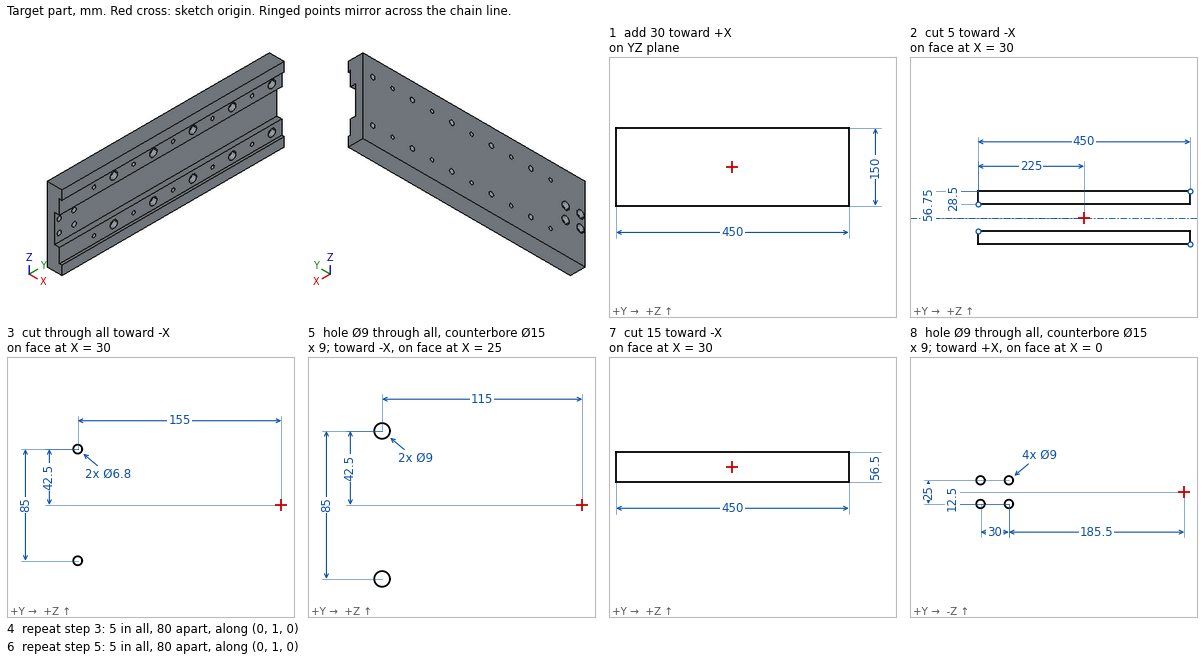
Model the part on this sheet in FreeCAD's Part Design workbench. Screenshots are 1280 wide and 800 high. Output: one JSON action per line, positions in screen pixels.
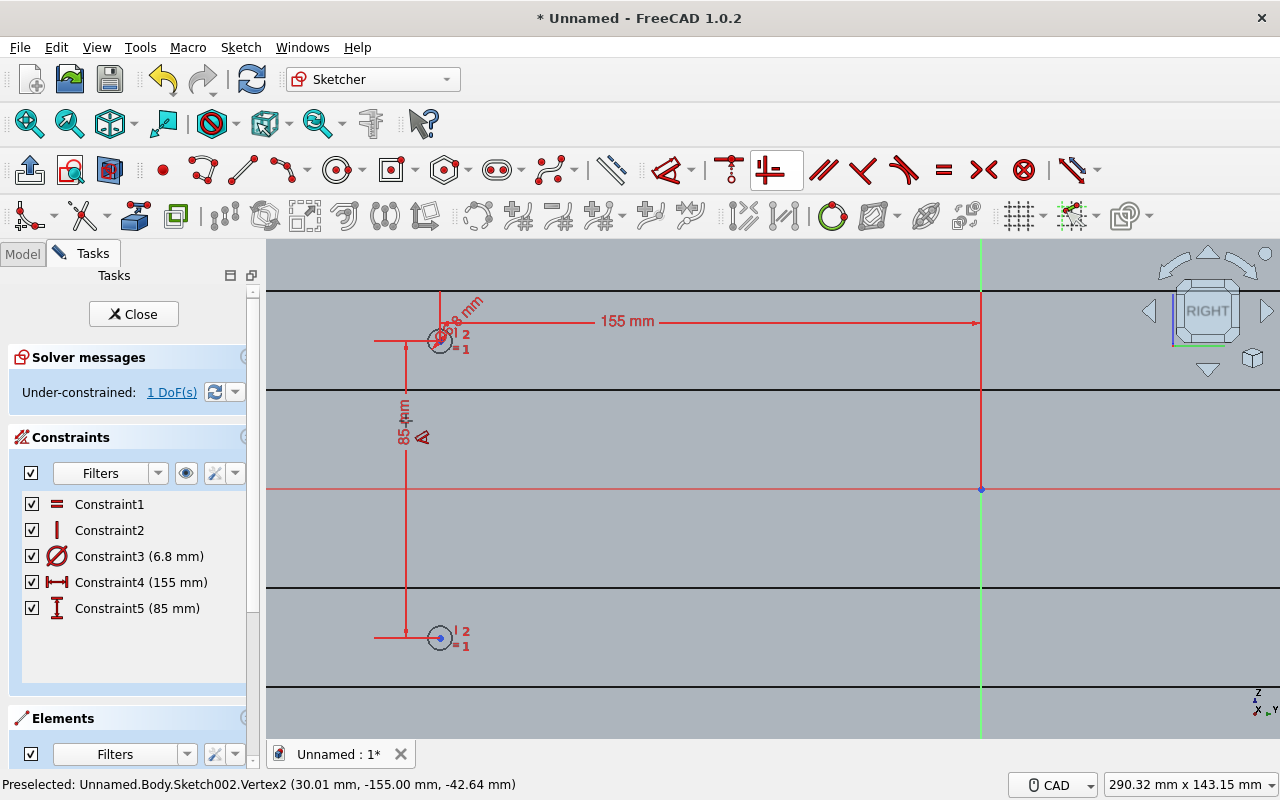
{"action": "left_click", "coordinate": [440, 341]}
{"action": "left_click", "coordinate": [1015, 415]}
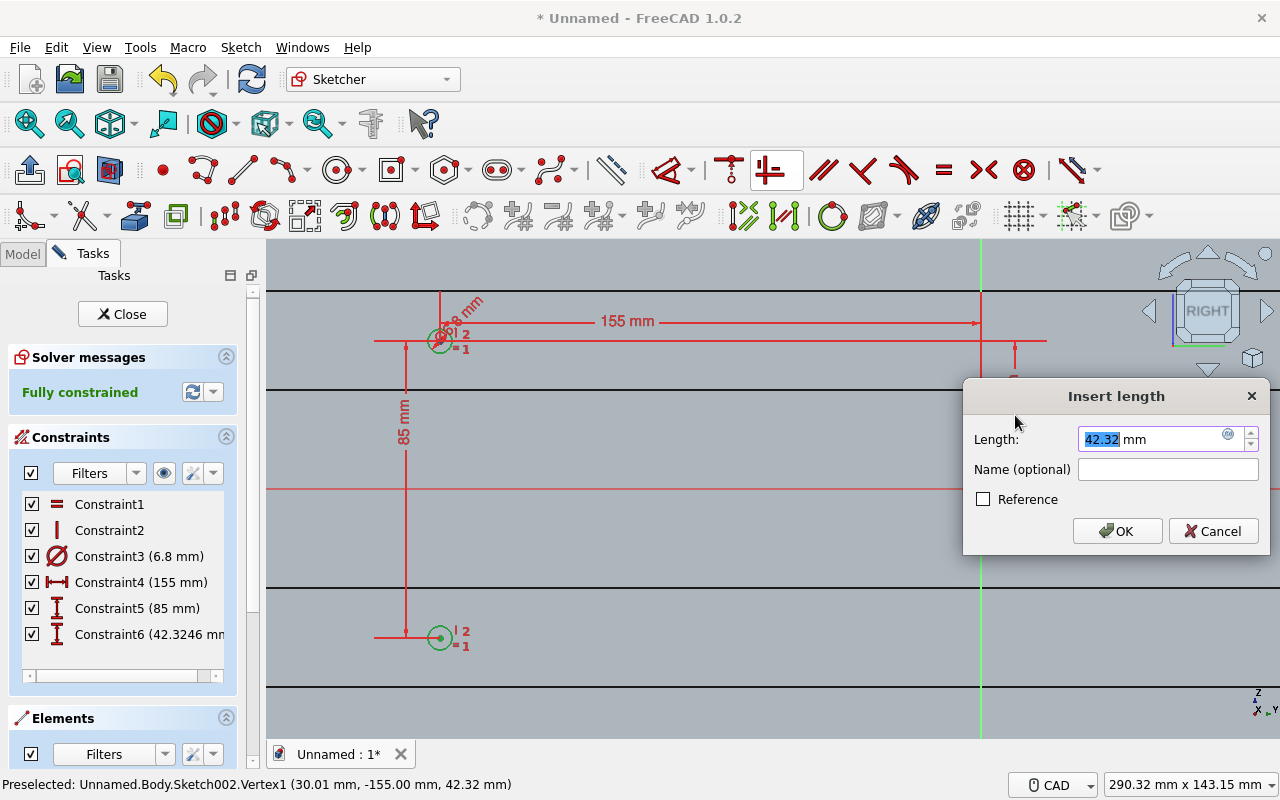
{"action": "type", "text": "42.5"}
{"action": "key", "text": "Return"}
{"action": "key", "text": "Escape"}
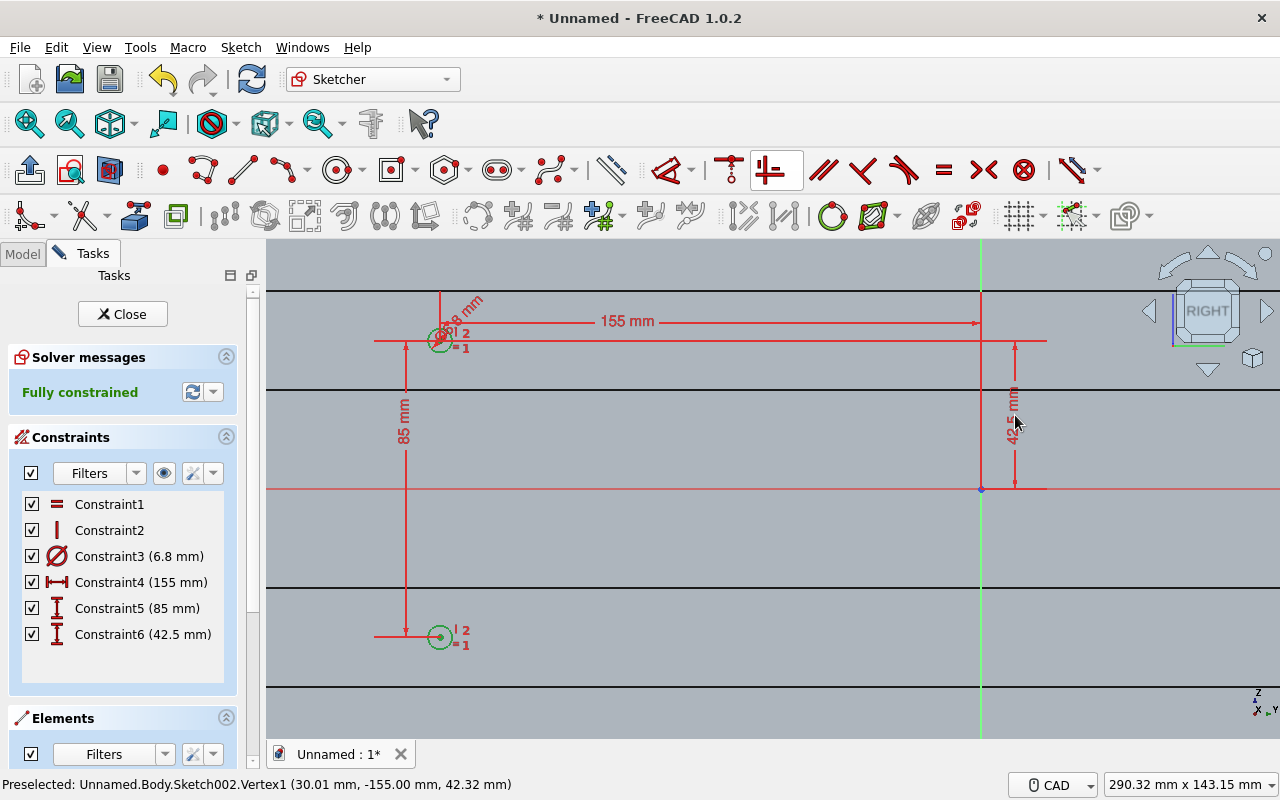
{"action": "left_click", "coordinate": [123, 314]}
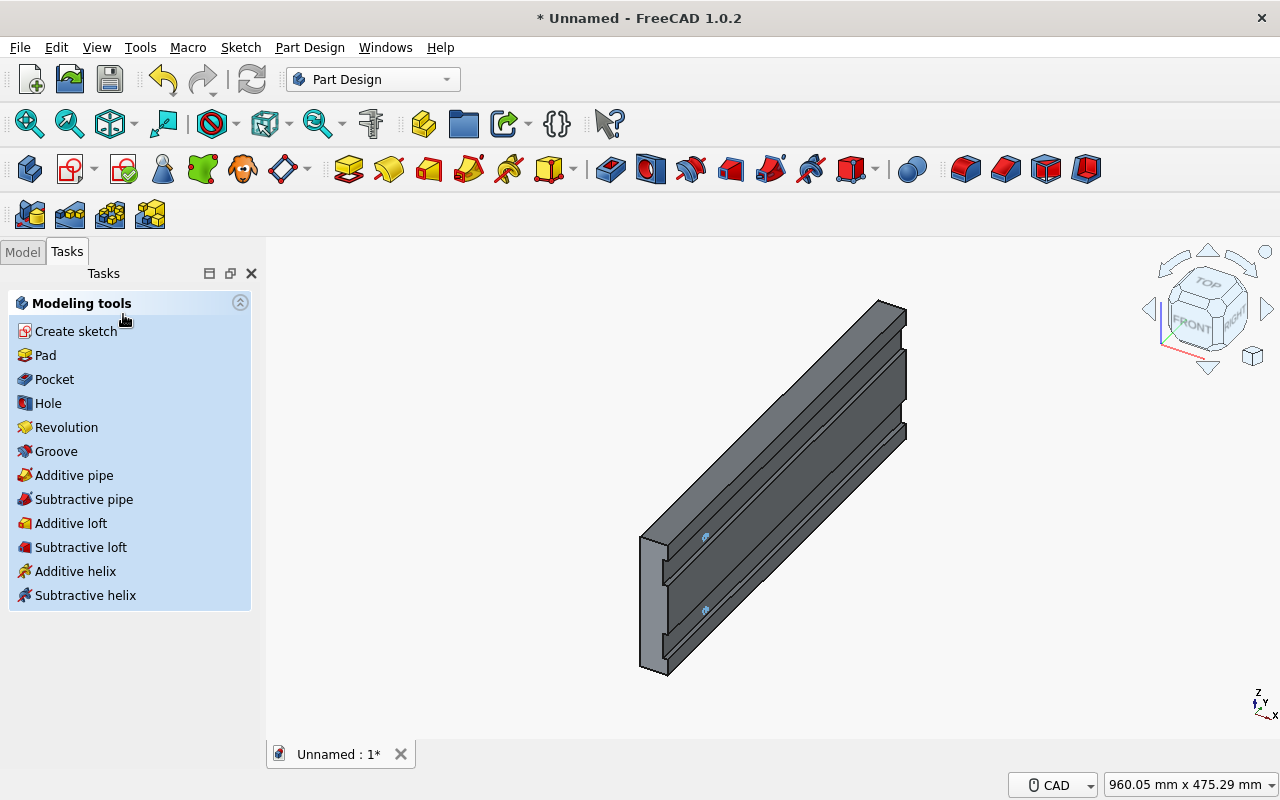
{"action": "left_click", "coordinate": [612, 170]}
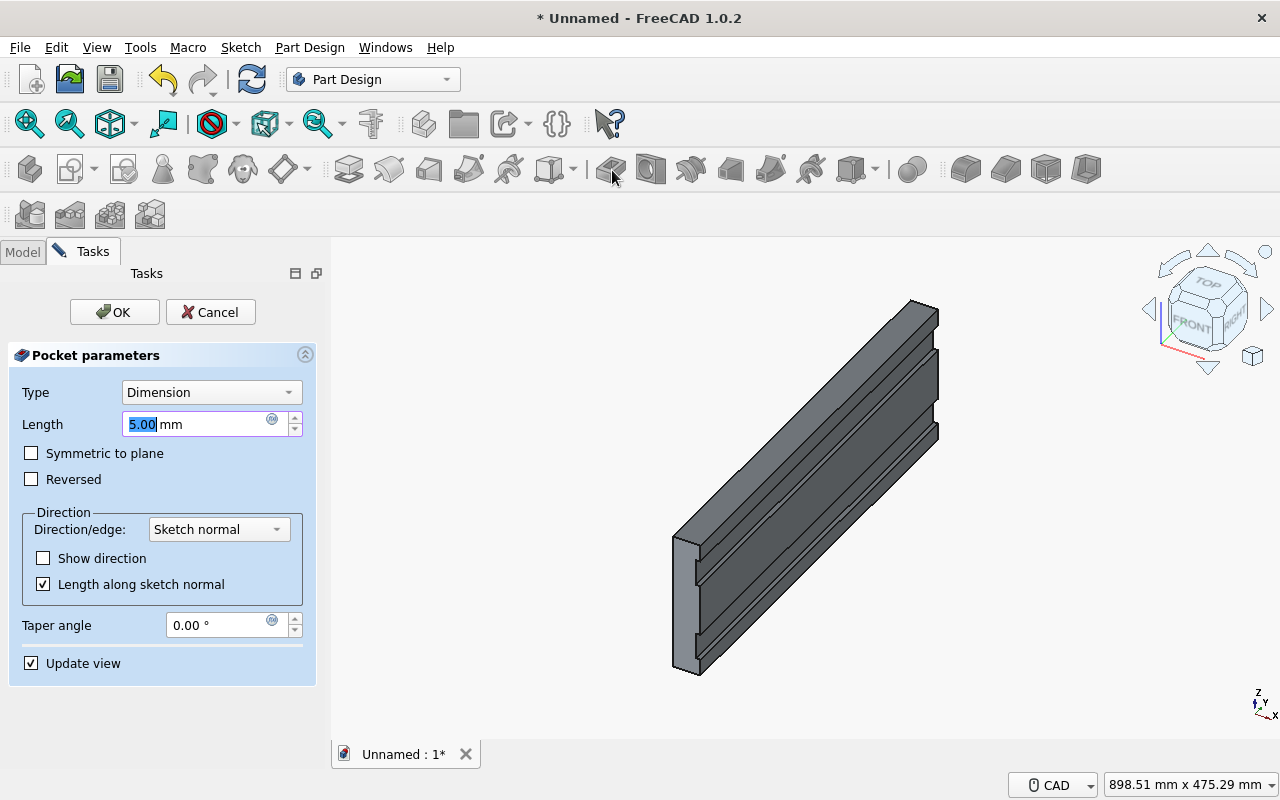
{"action": "left_click", "coordinate": [212, 392]}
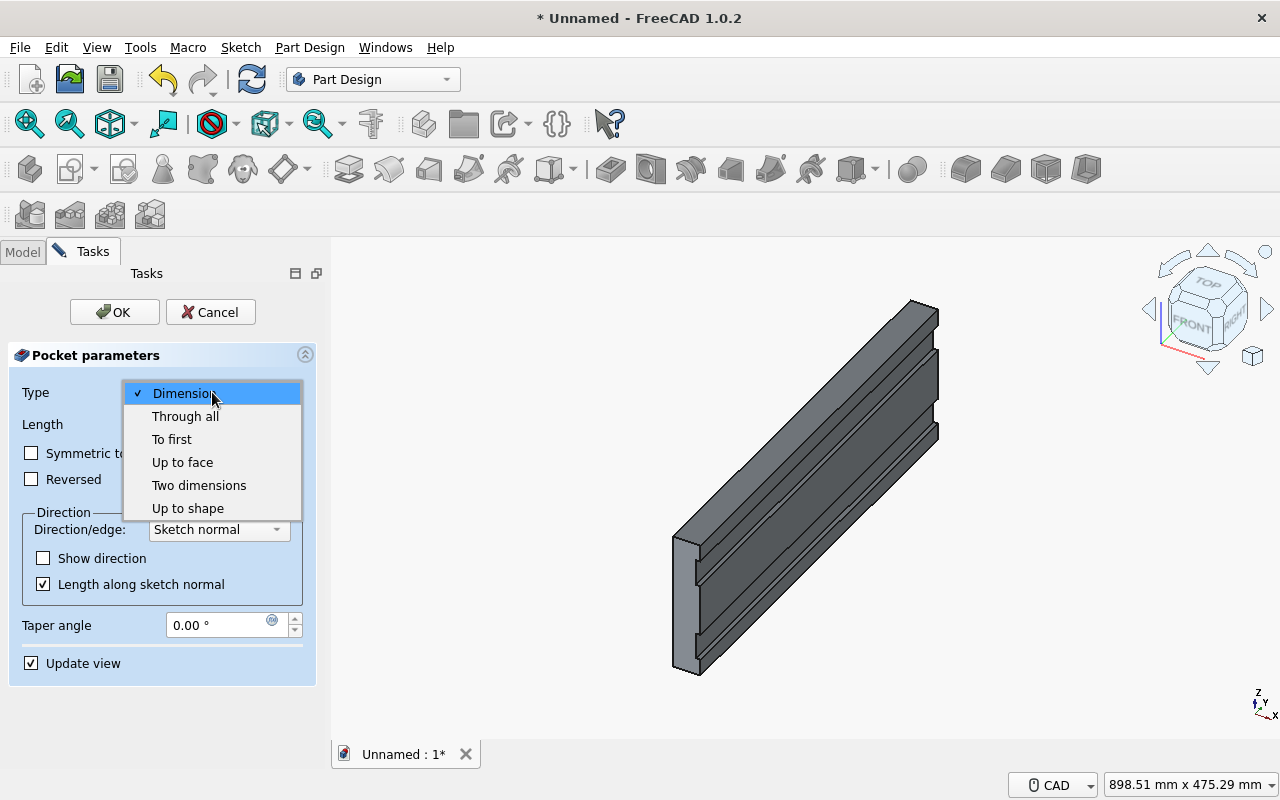
{"action": "left_click", "coordinate": [212, 416]}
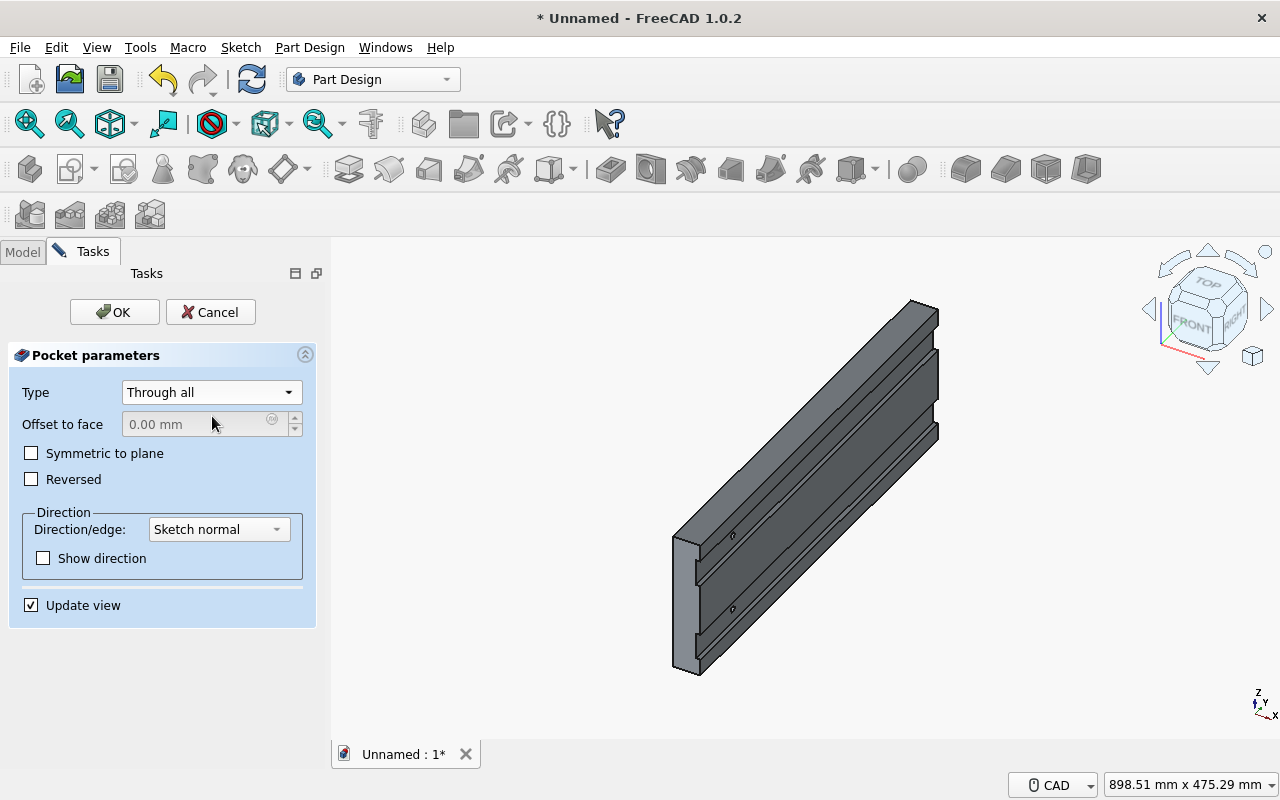
{"action": "left_click", "coordinate": [115, 312]}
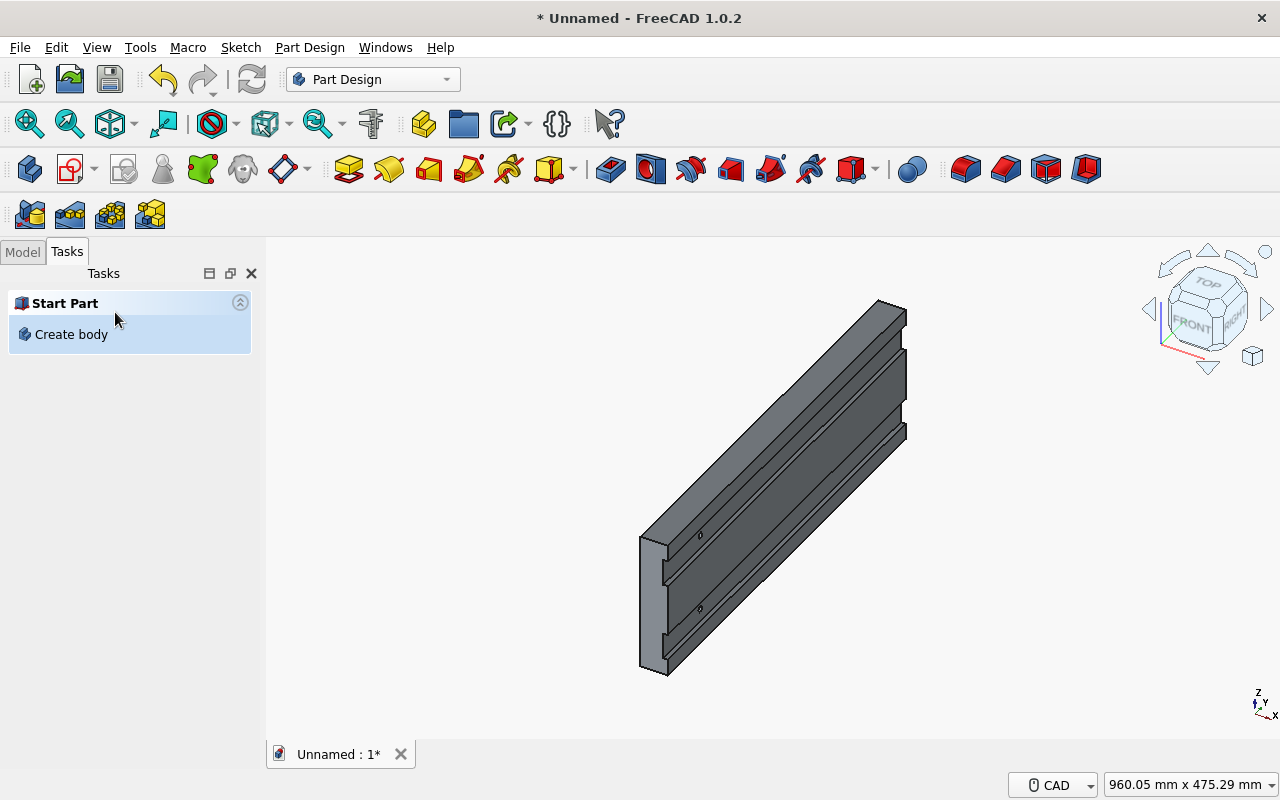
{"action": "left_click", "coordinate": [23, 251]}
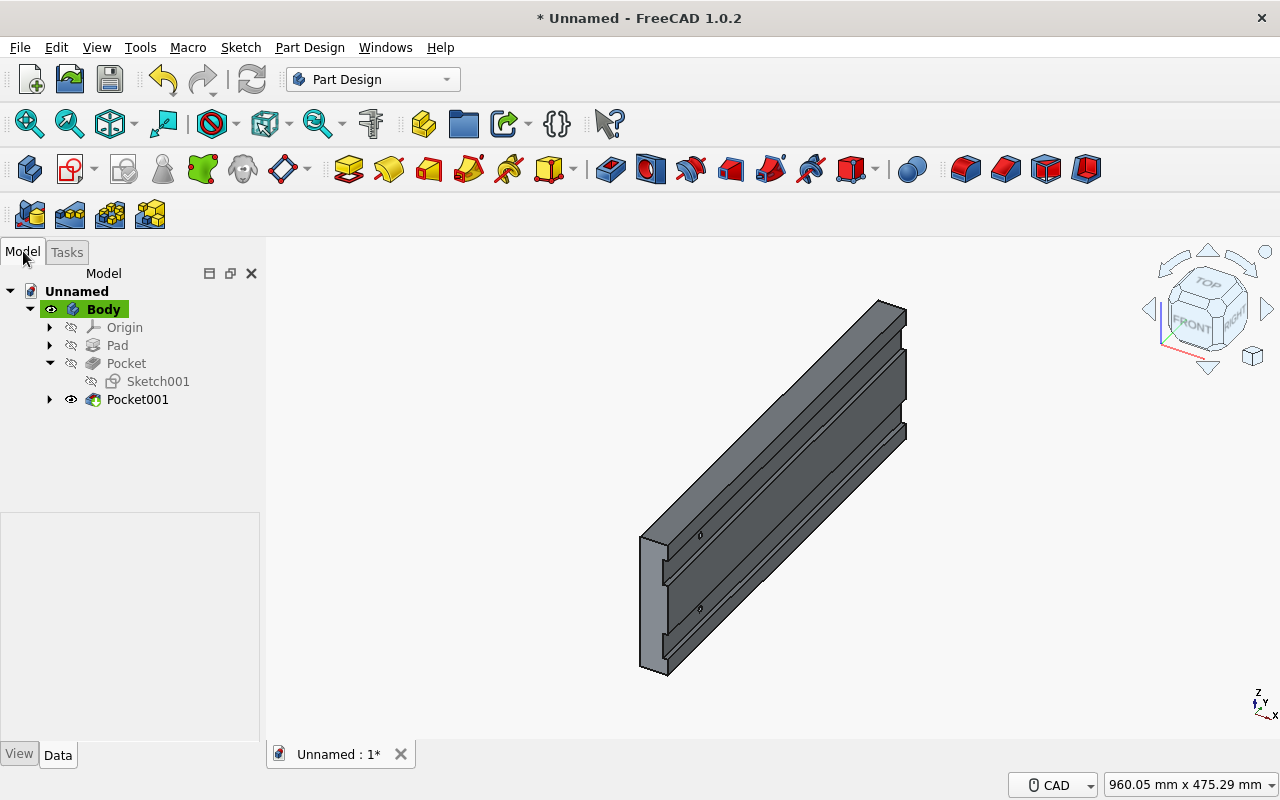
{"action": "left_click", "coordinate": [116, 399]}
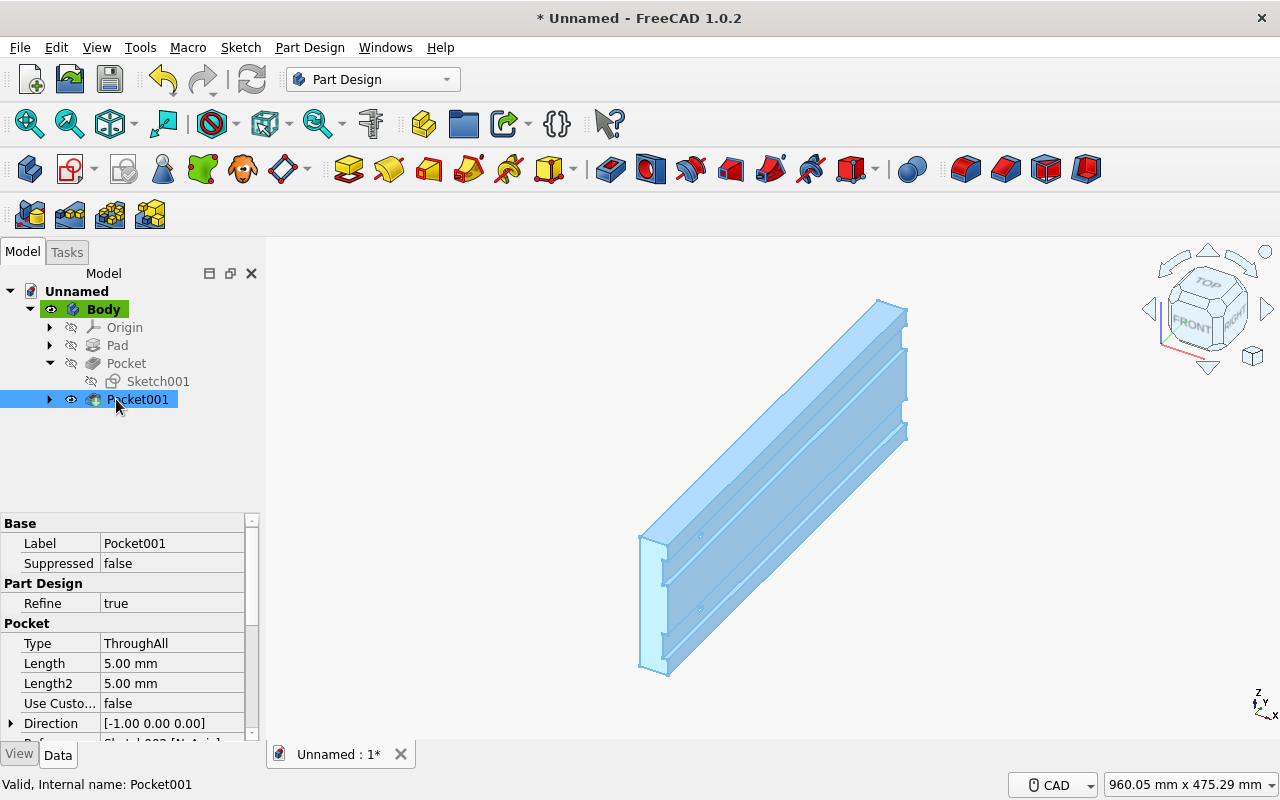
{"action": "left_click", "coordinate": [70, 214]}